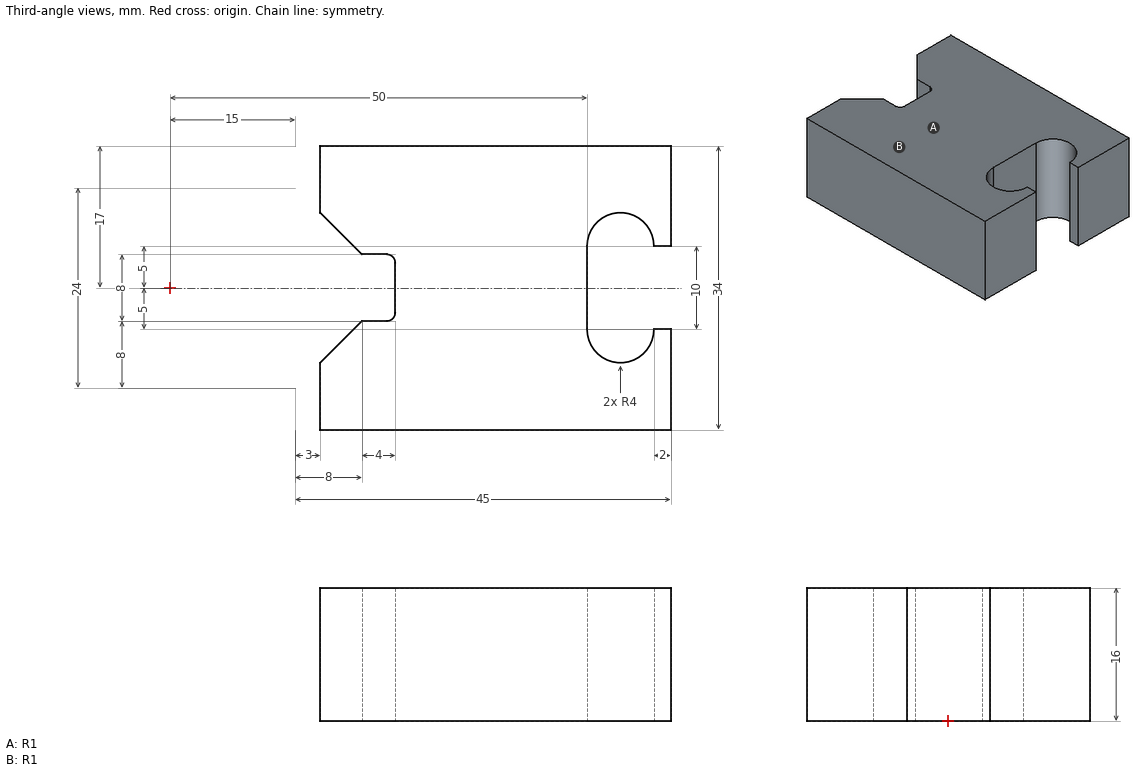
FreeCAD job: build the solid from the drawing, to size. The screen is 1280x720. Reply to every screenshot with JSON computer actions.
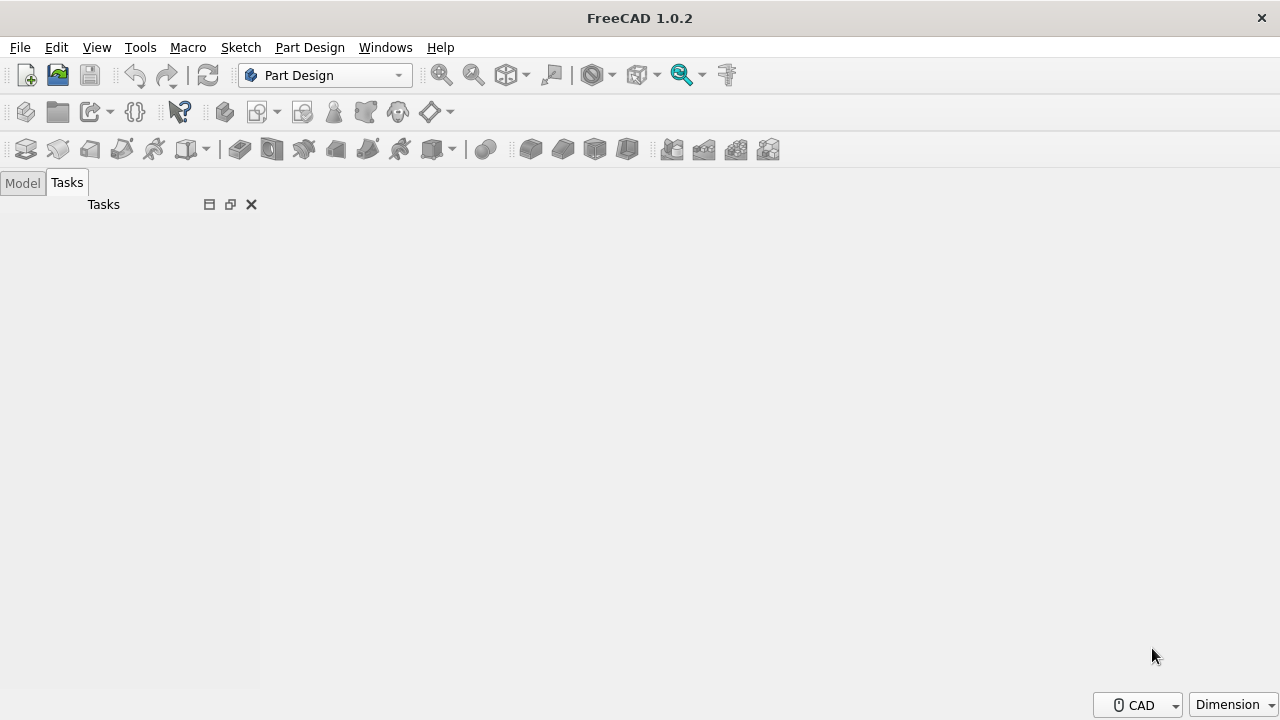
{"action": "left_click", "coordinate": [26, 76]}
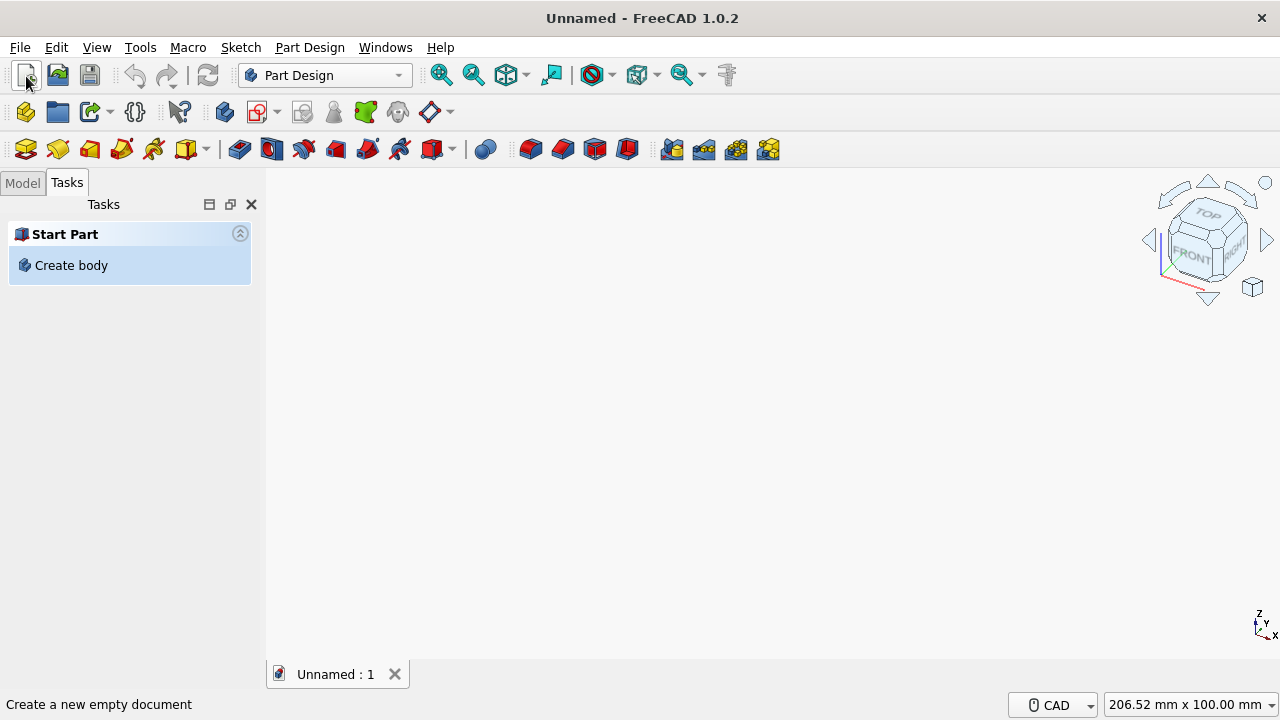
{"action": "left_click", "coordinate": [258, 112]}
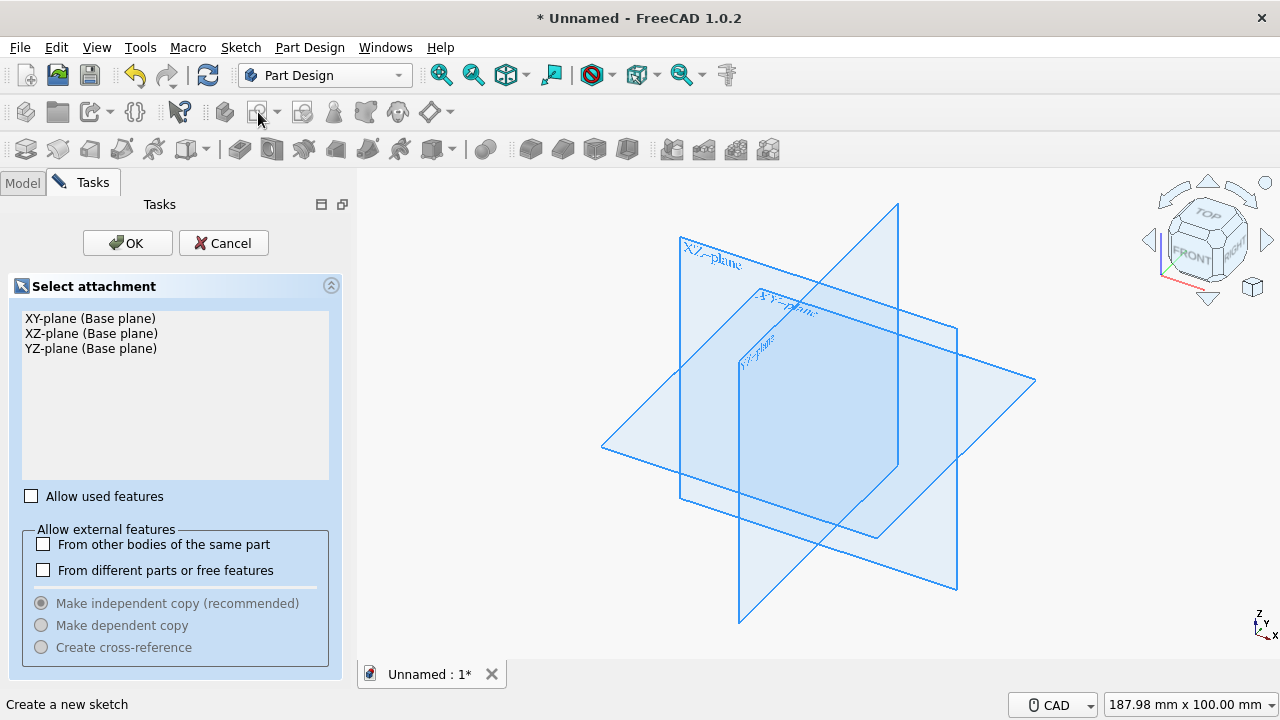
{"action": "left_click", "coordinate": [82, 318]}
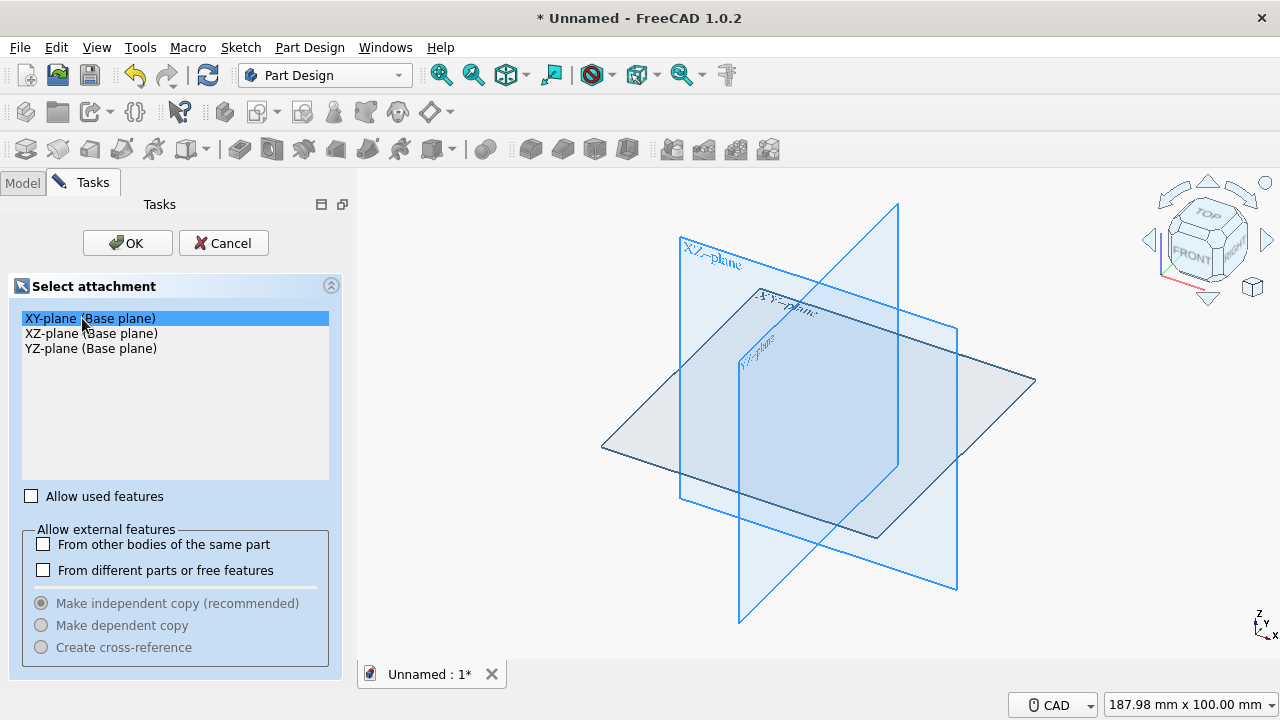
{"action": "left_click", "coordinate": [128, 243]}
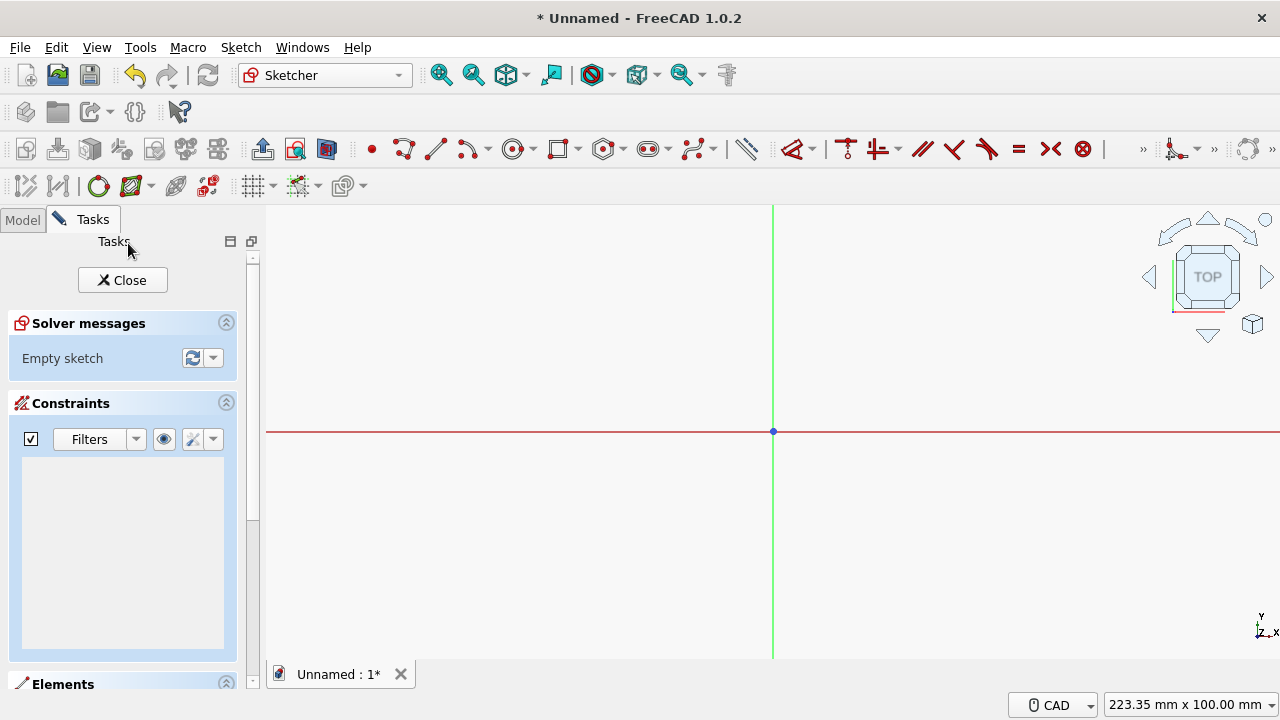
{"action": "scroll", "coordinate": [1115, 432], "scroll_direction": "up", "scroll_amount": 3}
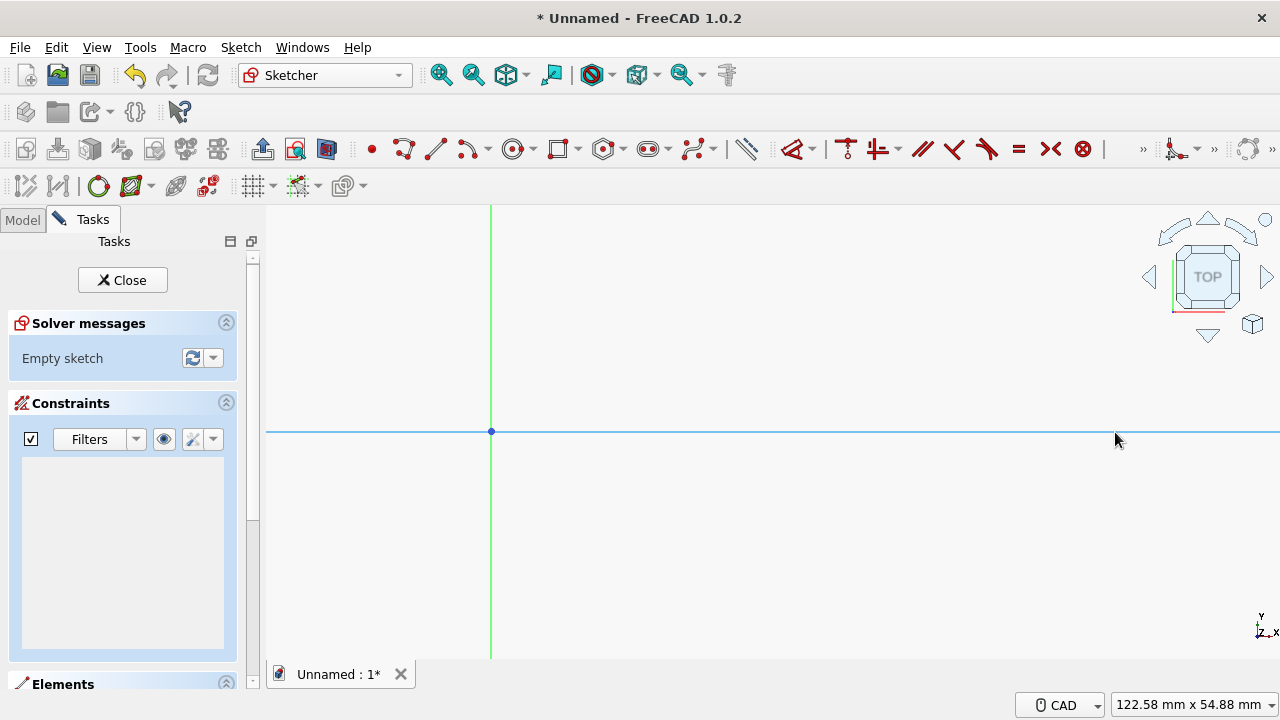
{"action": "left_click", "coordinate": [558, 150]}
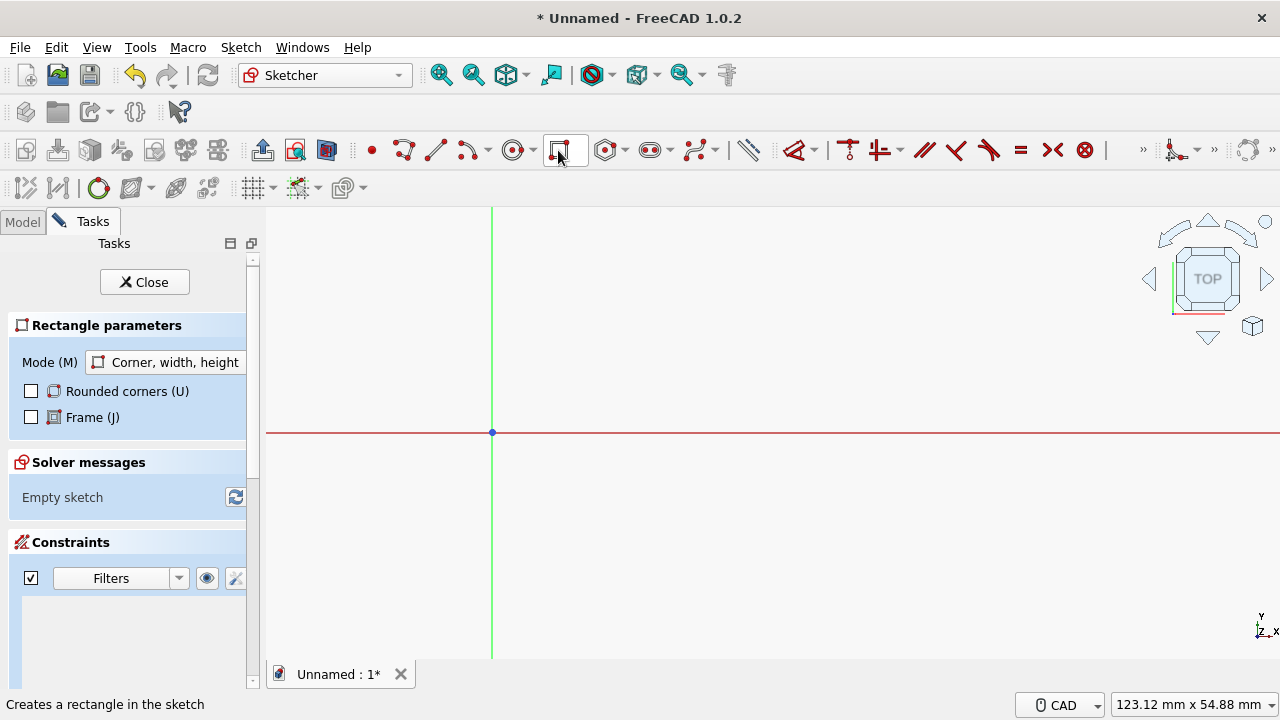
{"action": "left_click", "coordinate": [616, 293]}
{"action": "mouse_move", "coordinate": [987, 573]}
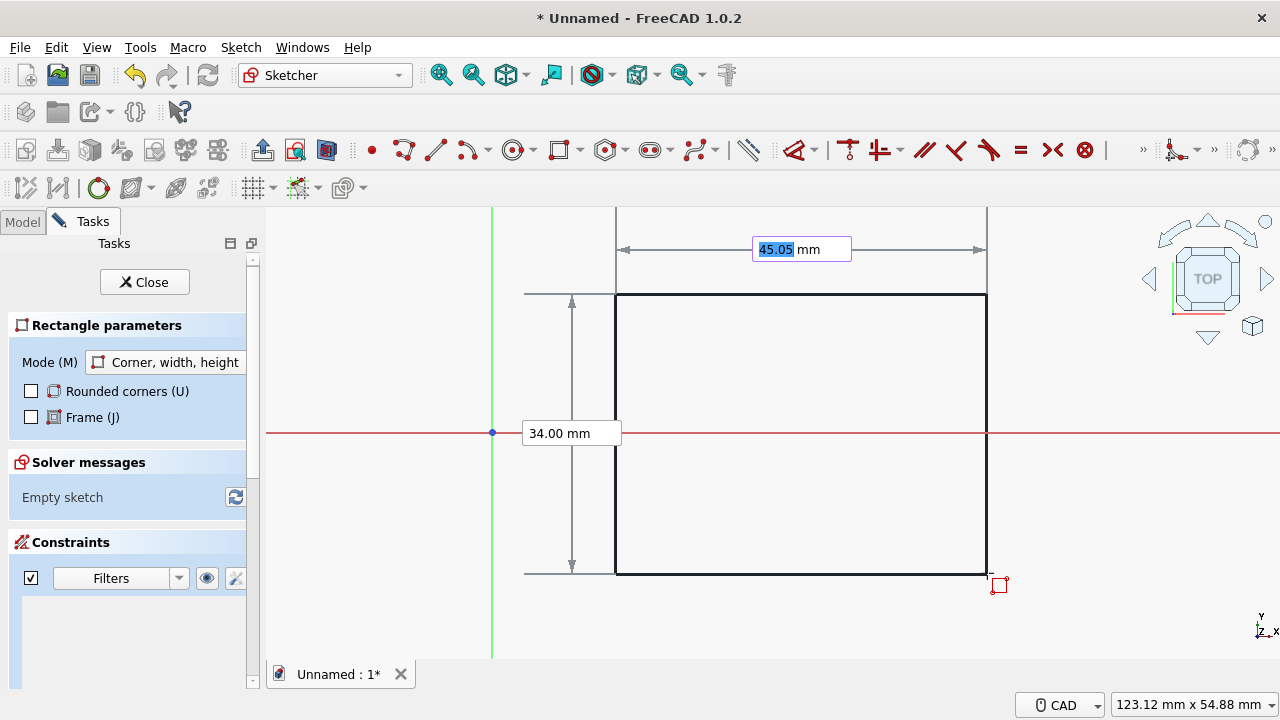
{"action": "type", "text": "45"}
{"action": "key", "text": "Tab"}
{"action": "type", "text": "34"}
{"action": "key", "text": "Return"}
{"action": "key", "text": "Escape"}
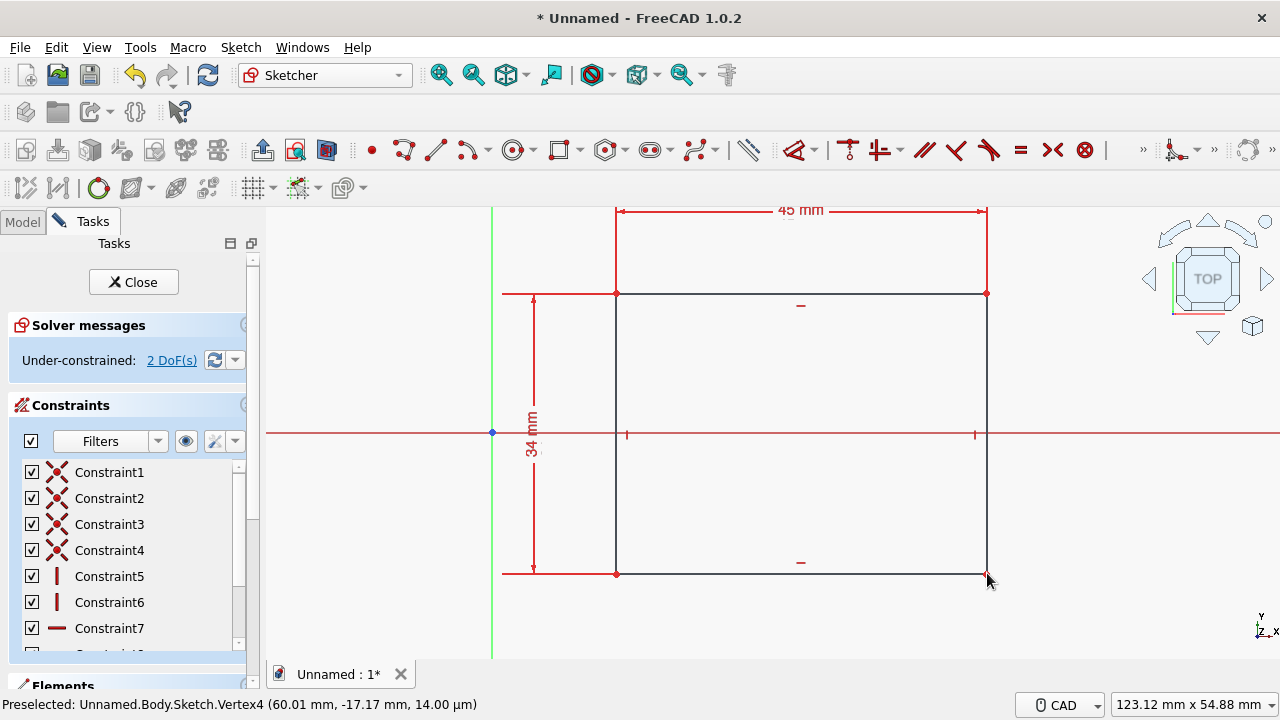
{"action": "left_click", "coordinate": [616, 294]}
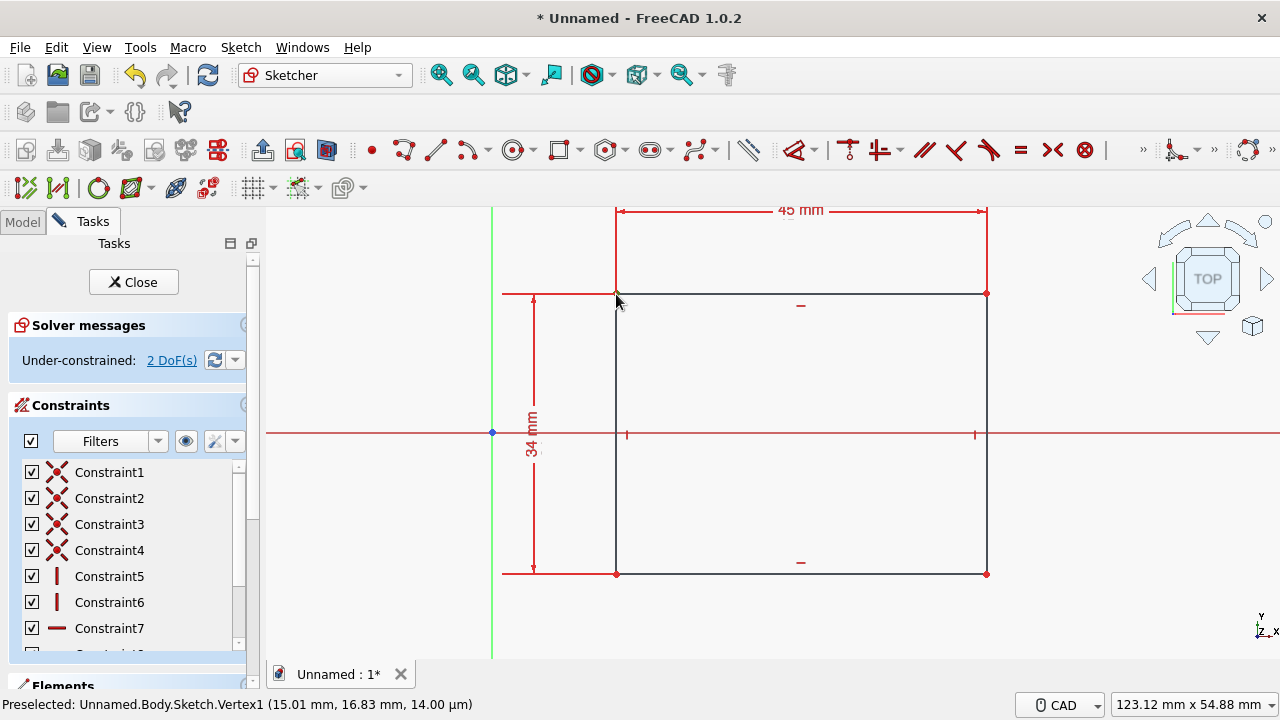
{"action": "left_click", "coordinate": [816, 150]}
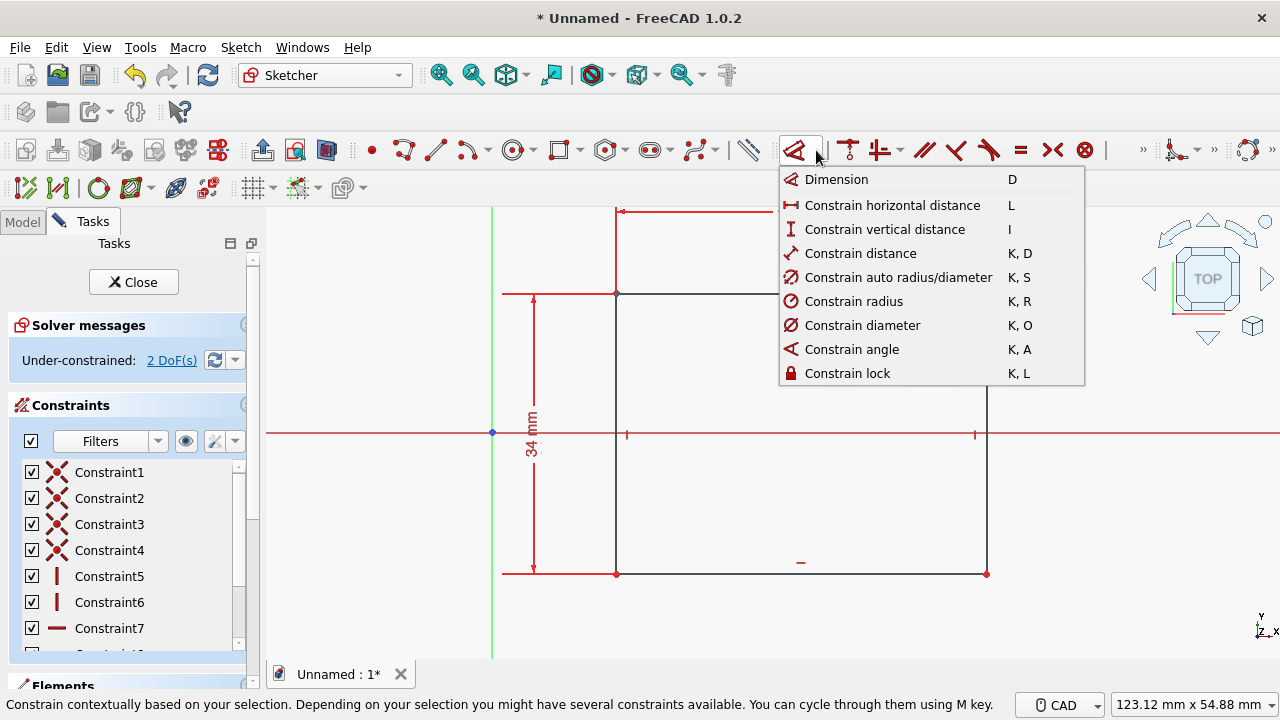
{"action": "left_click", "coordinate": [932, 205]}